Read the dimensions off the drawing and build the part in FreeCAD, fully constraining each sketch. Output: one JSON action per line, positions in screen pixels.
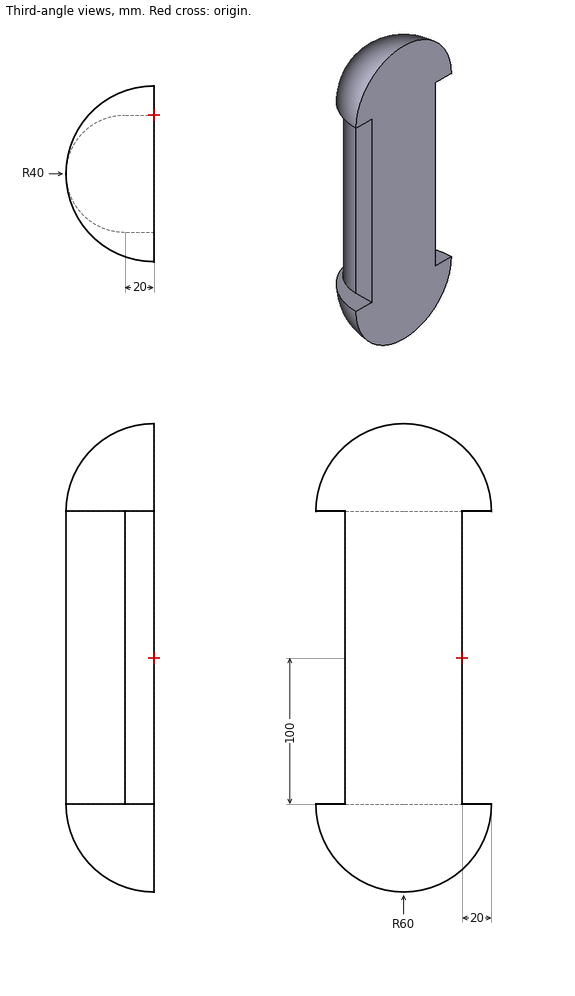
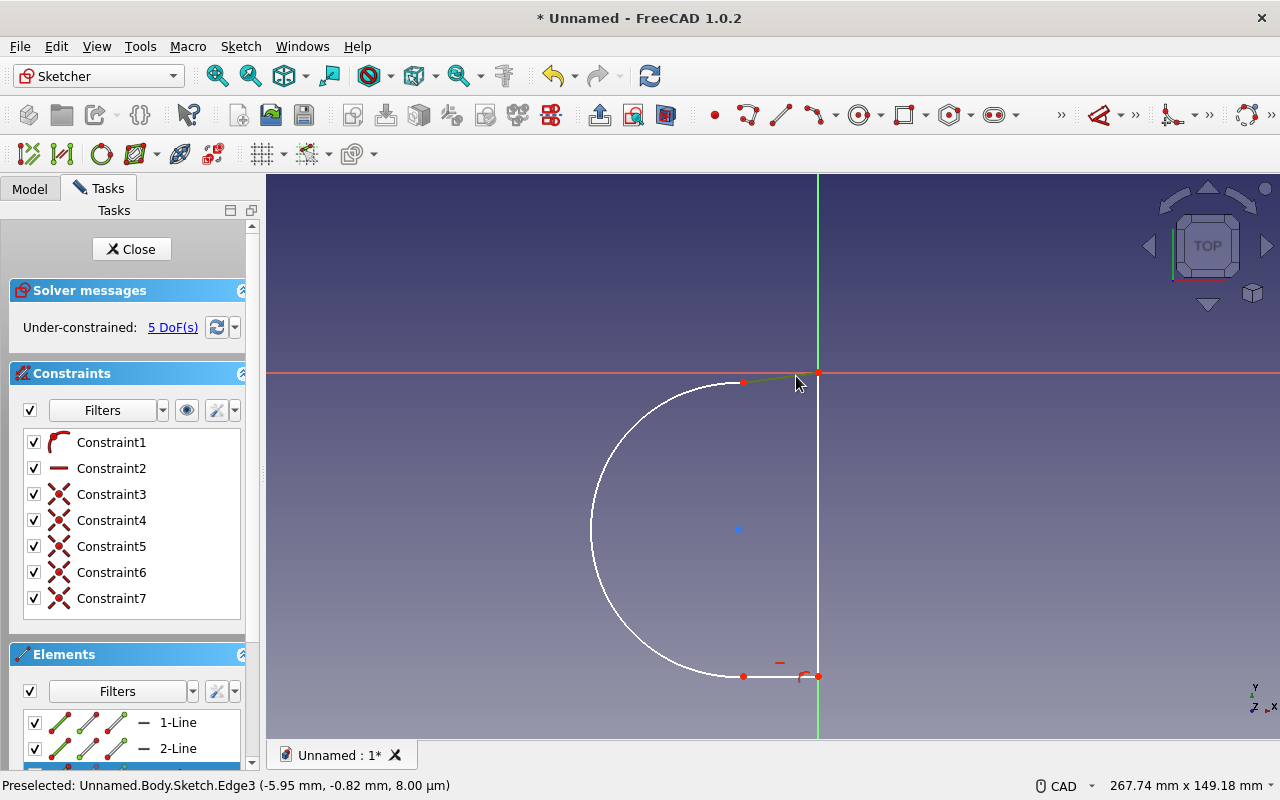
{"action": "left_click", "coordinate": [620, 442]}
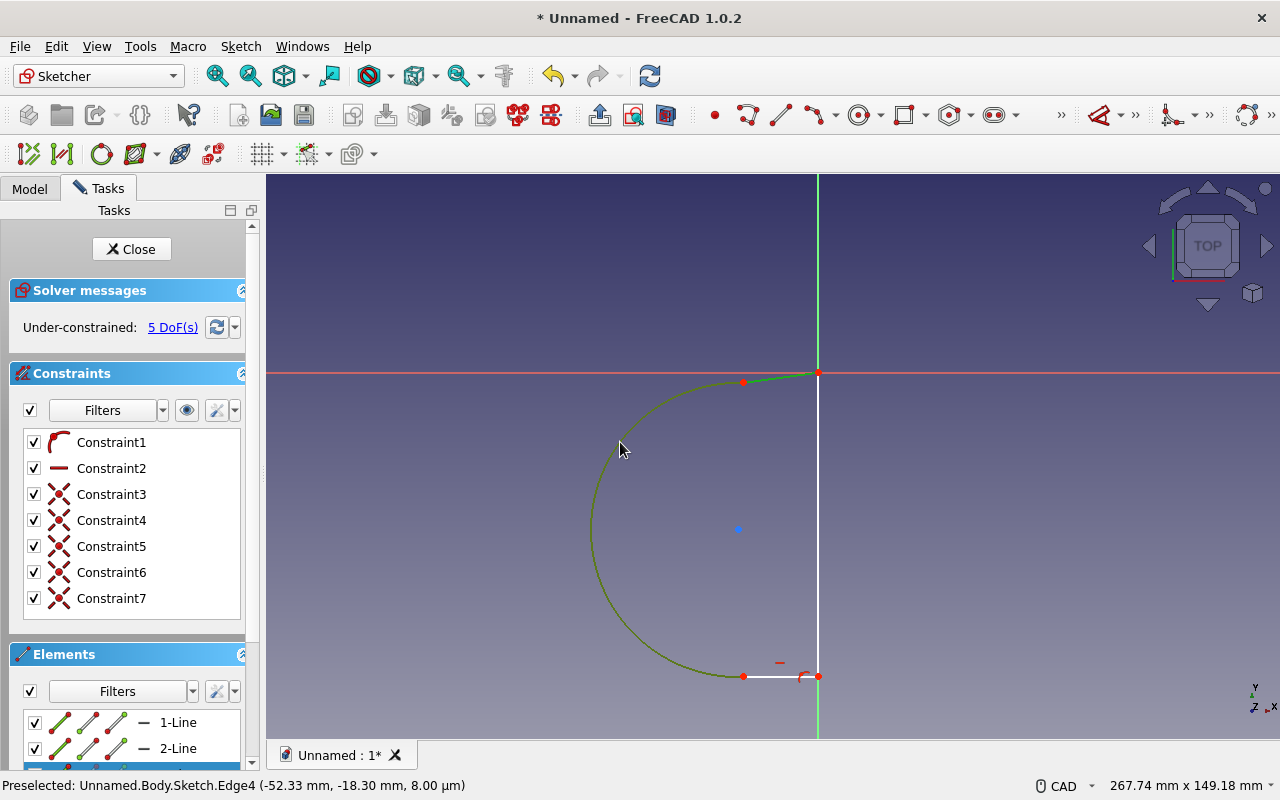
{"action": "key", "text": "t"}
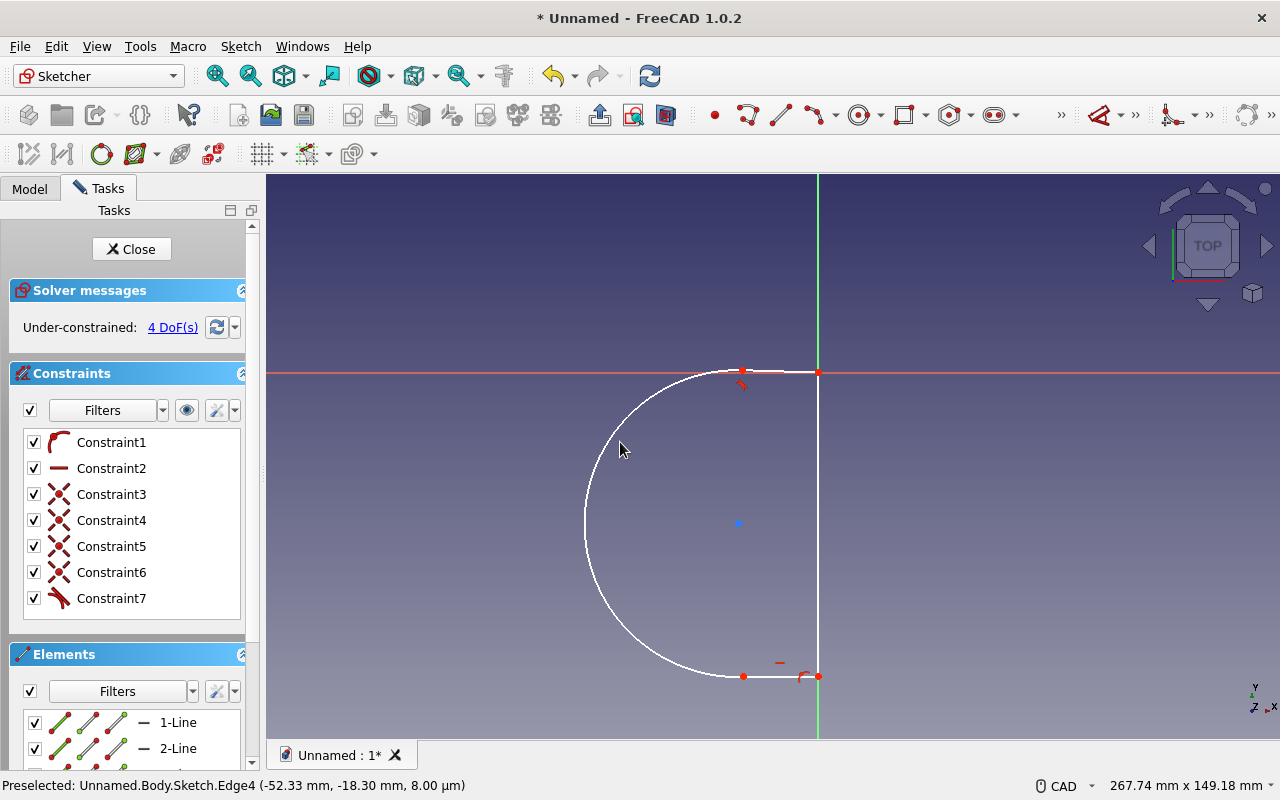
{"action": "left_click", "coordinate": [796, 372]}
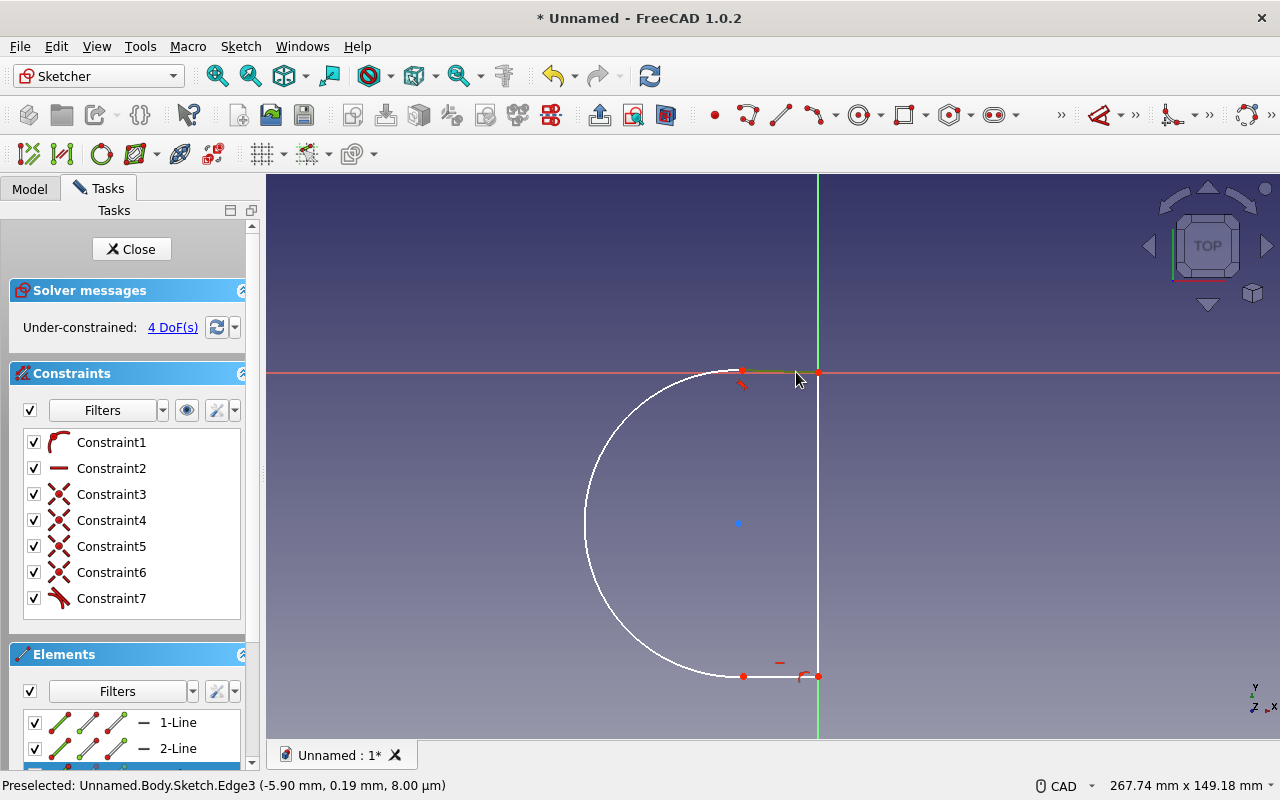
{"action": "key", "text": "h"}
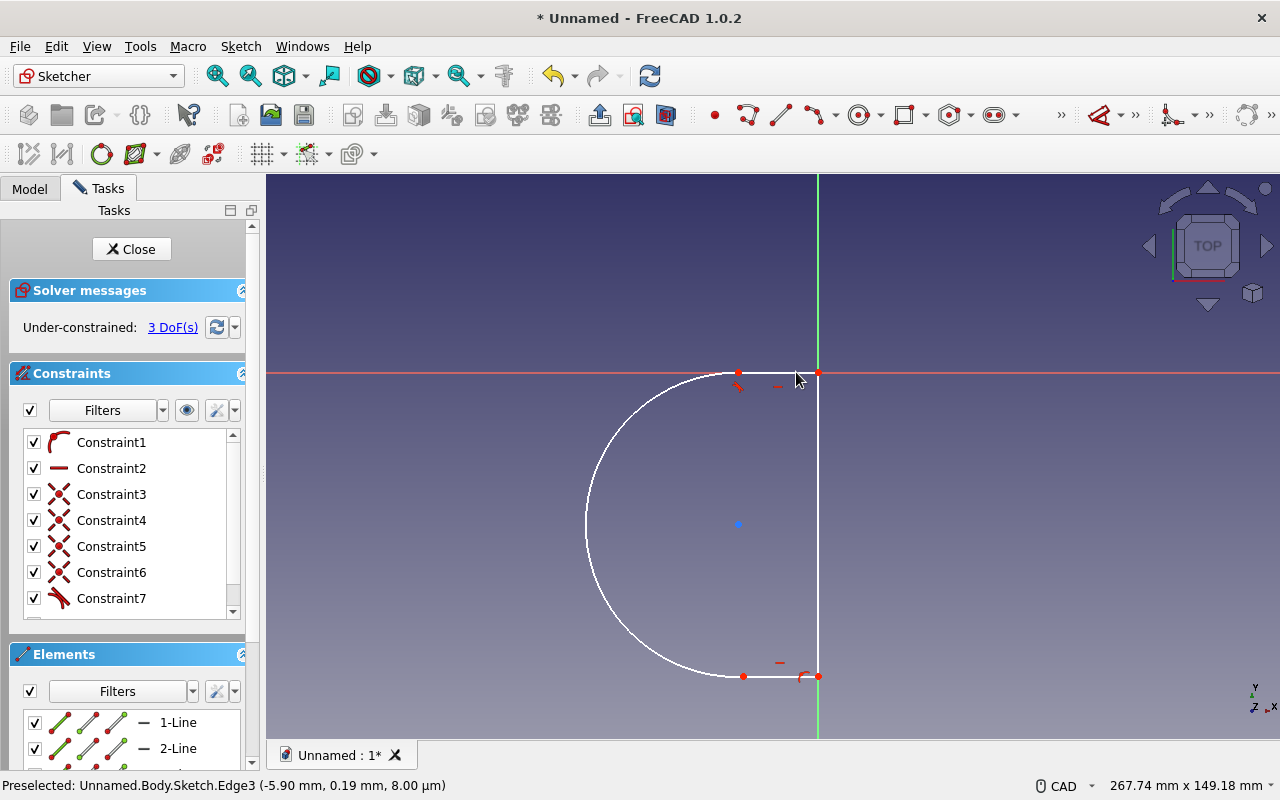
{"action": "key", "text": "d"}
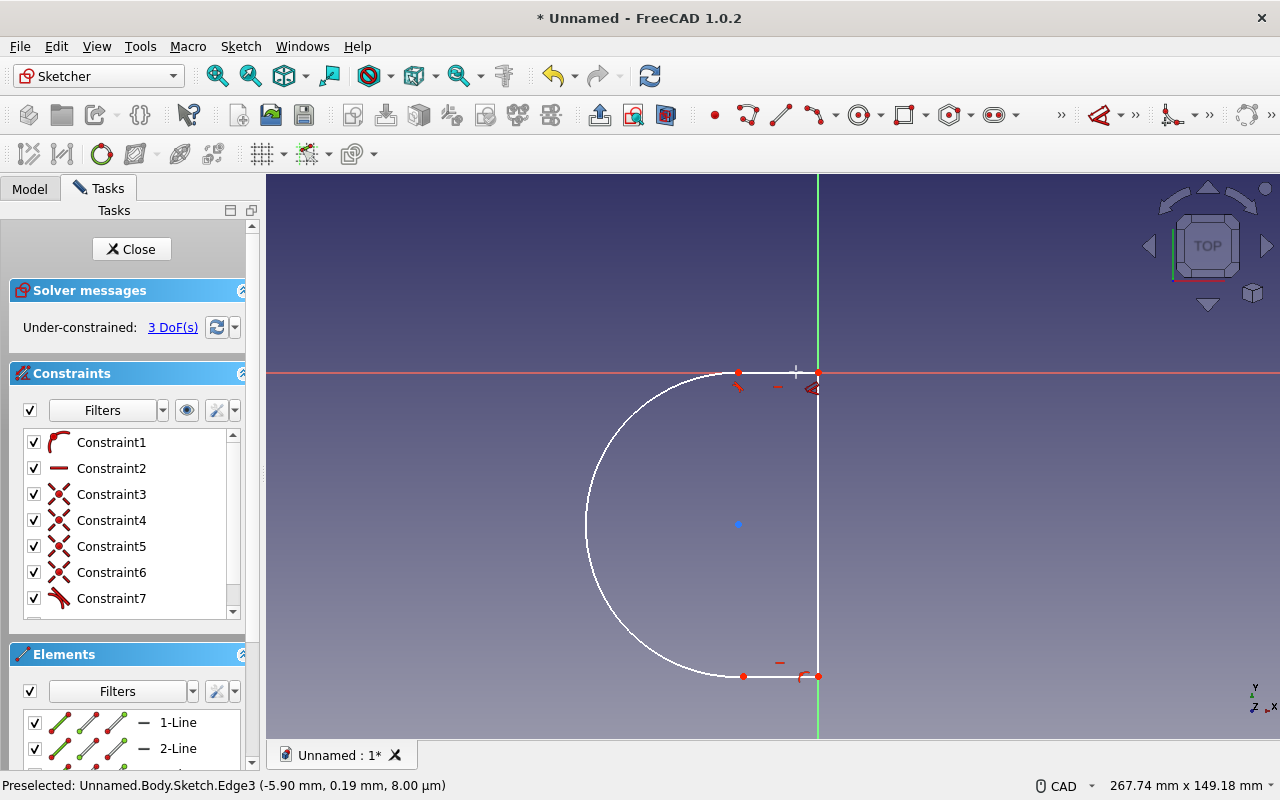
{"action": "left_click", "coordinate": [614, 437]}
{"action": "left_click", "coordinate": [588, 419]}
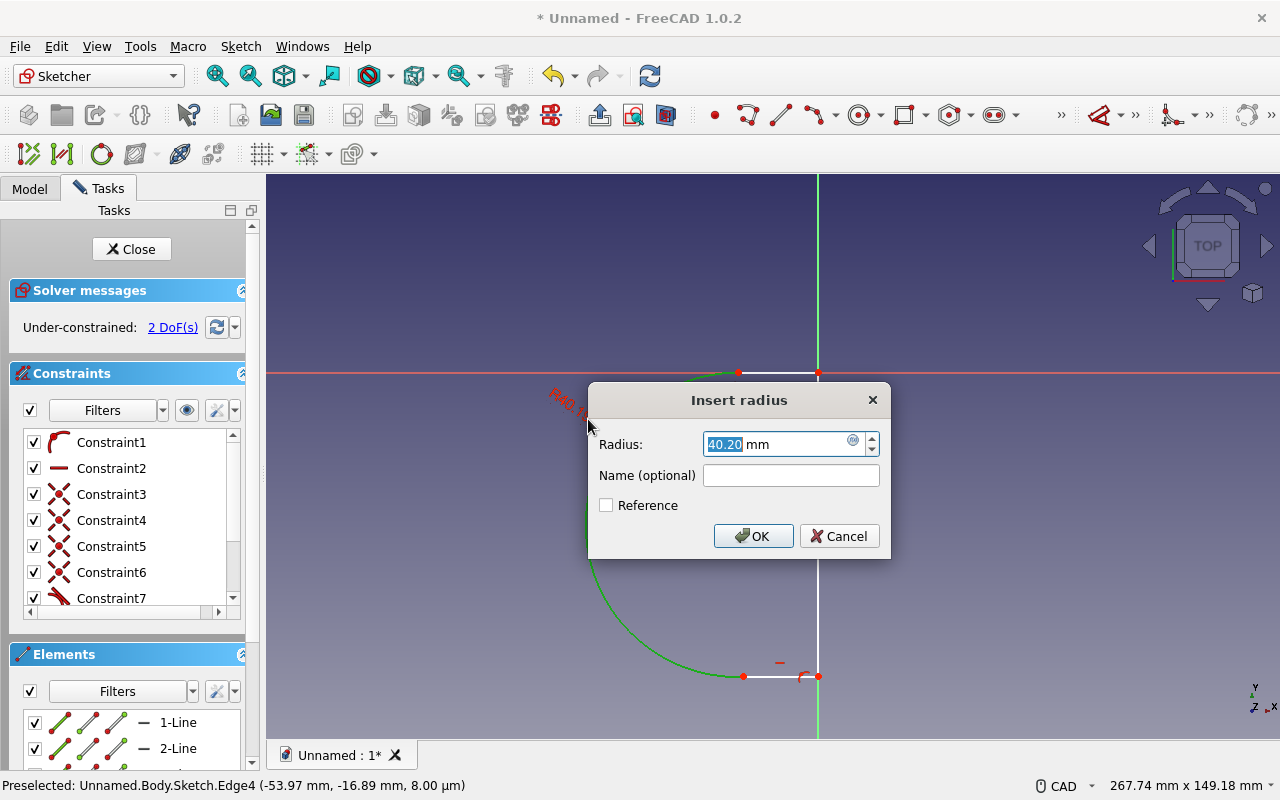
{"action": "type", "text": "40"}
{"action": "key", "text": "Return"}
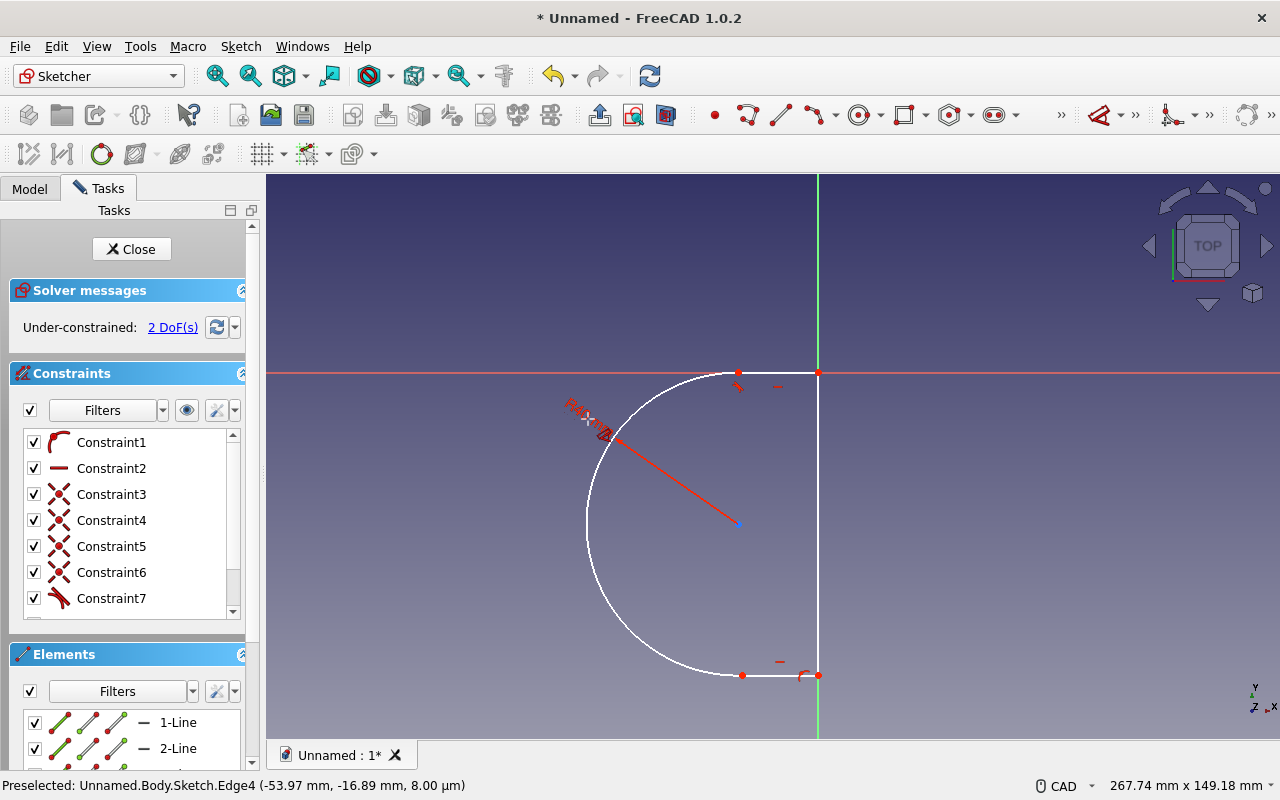
{"action": "left_click", "coordinate": [766, 676]}
{"action": "left_click", "coordinate": [781, 710]}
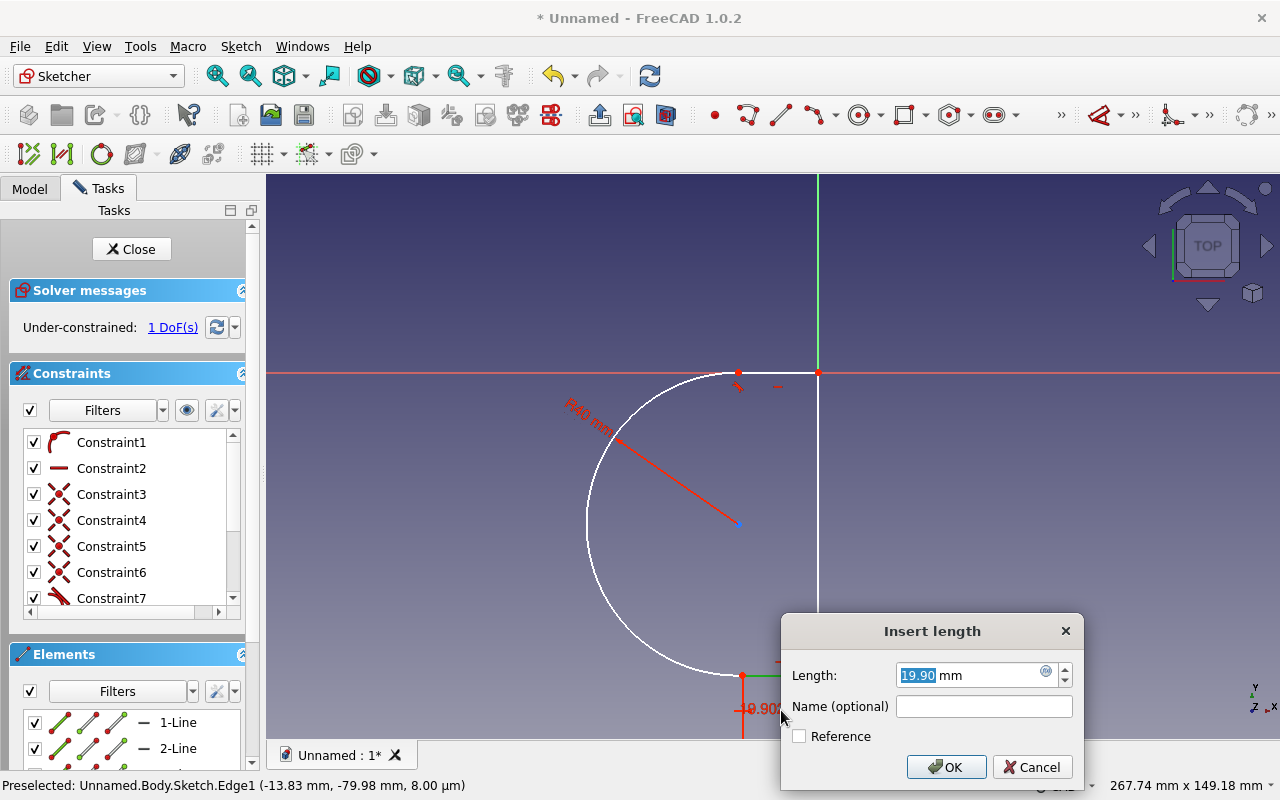
{"action": "type", "text": "20"}
{"action": "key", "text": "Return"}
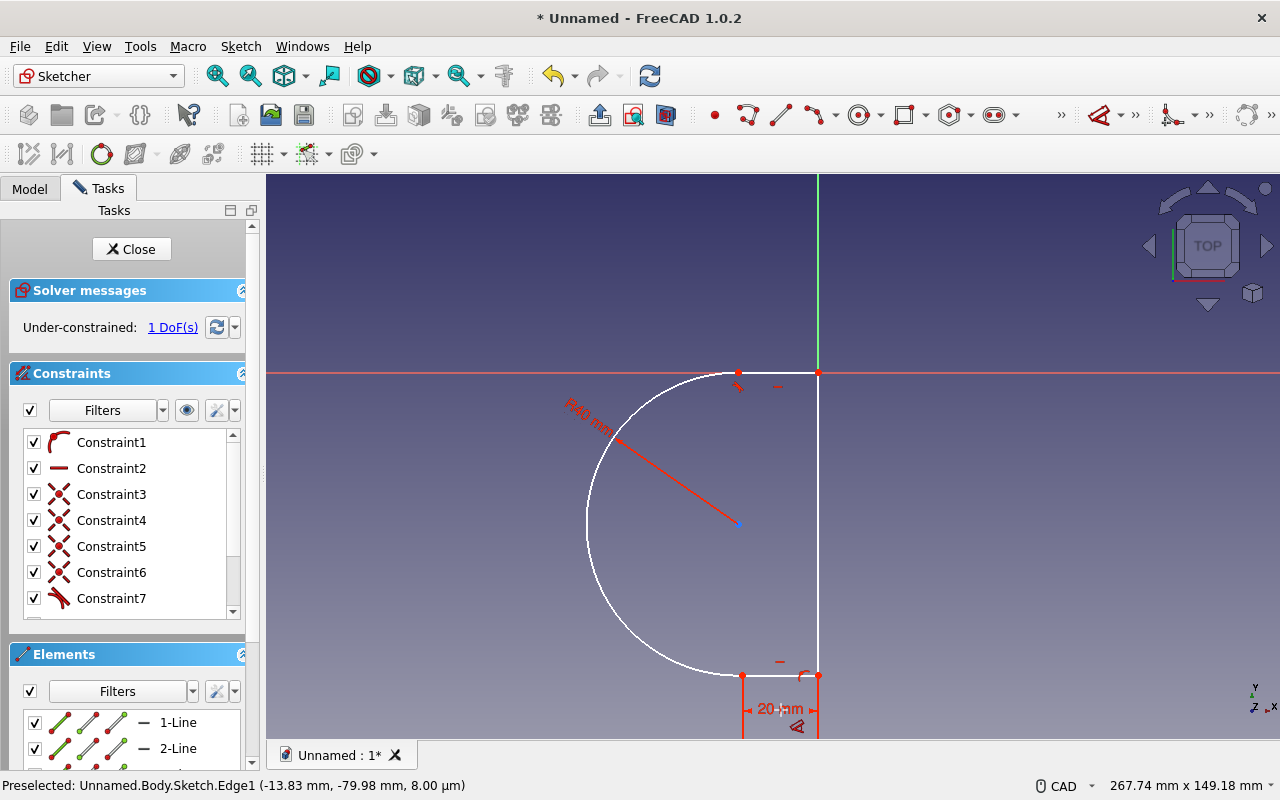
{"action": "left_click", "coordinate": [794, 373]}
{"action": "left_click", "coordinate": [778, 339]}